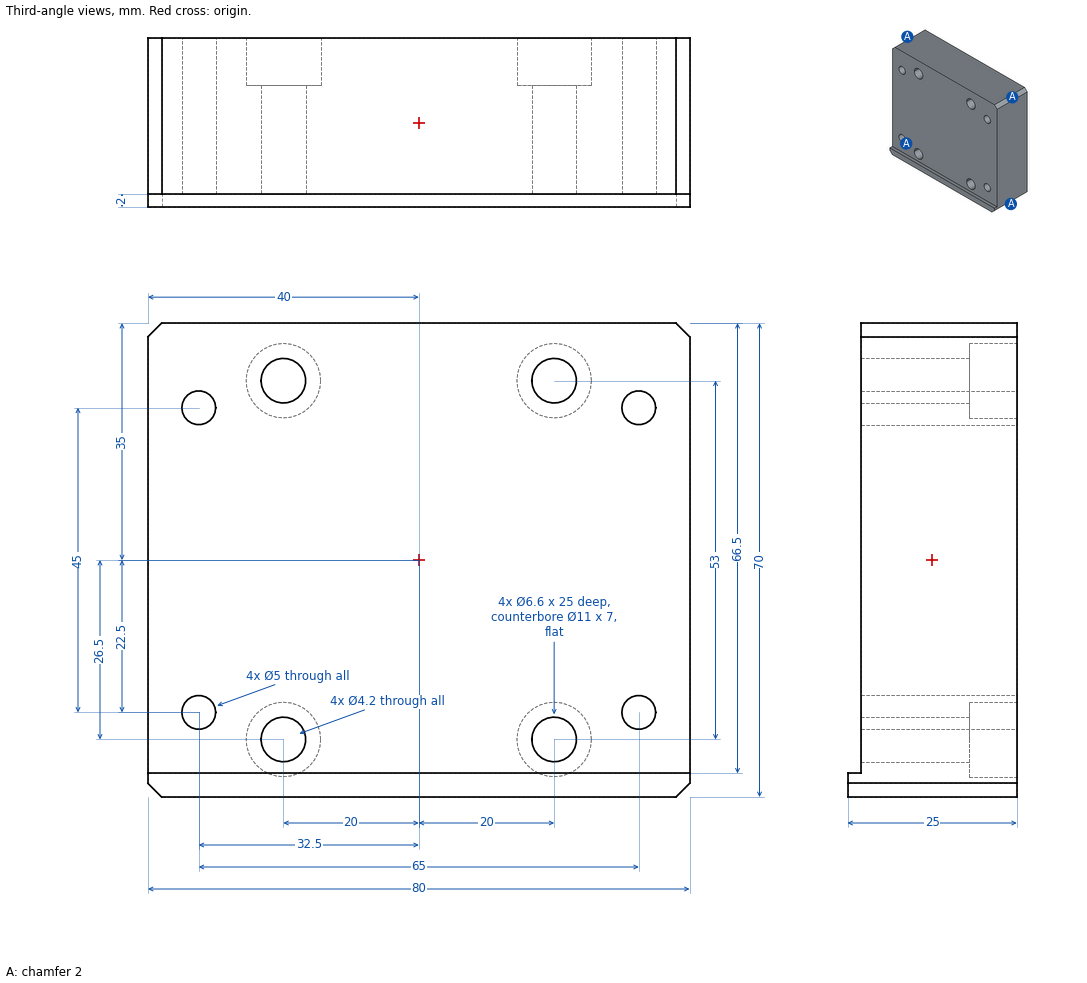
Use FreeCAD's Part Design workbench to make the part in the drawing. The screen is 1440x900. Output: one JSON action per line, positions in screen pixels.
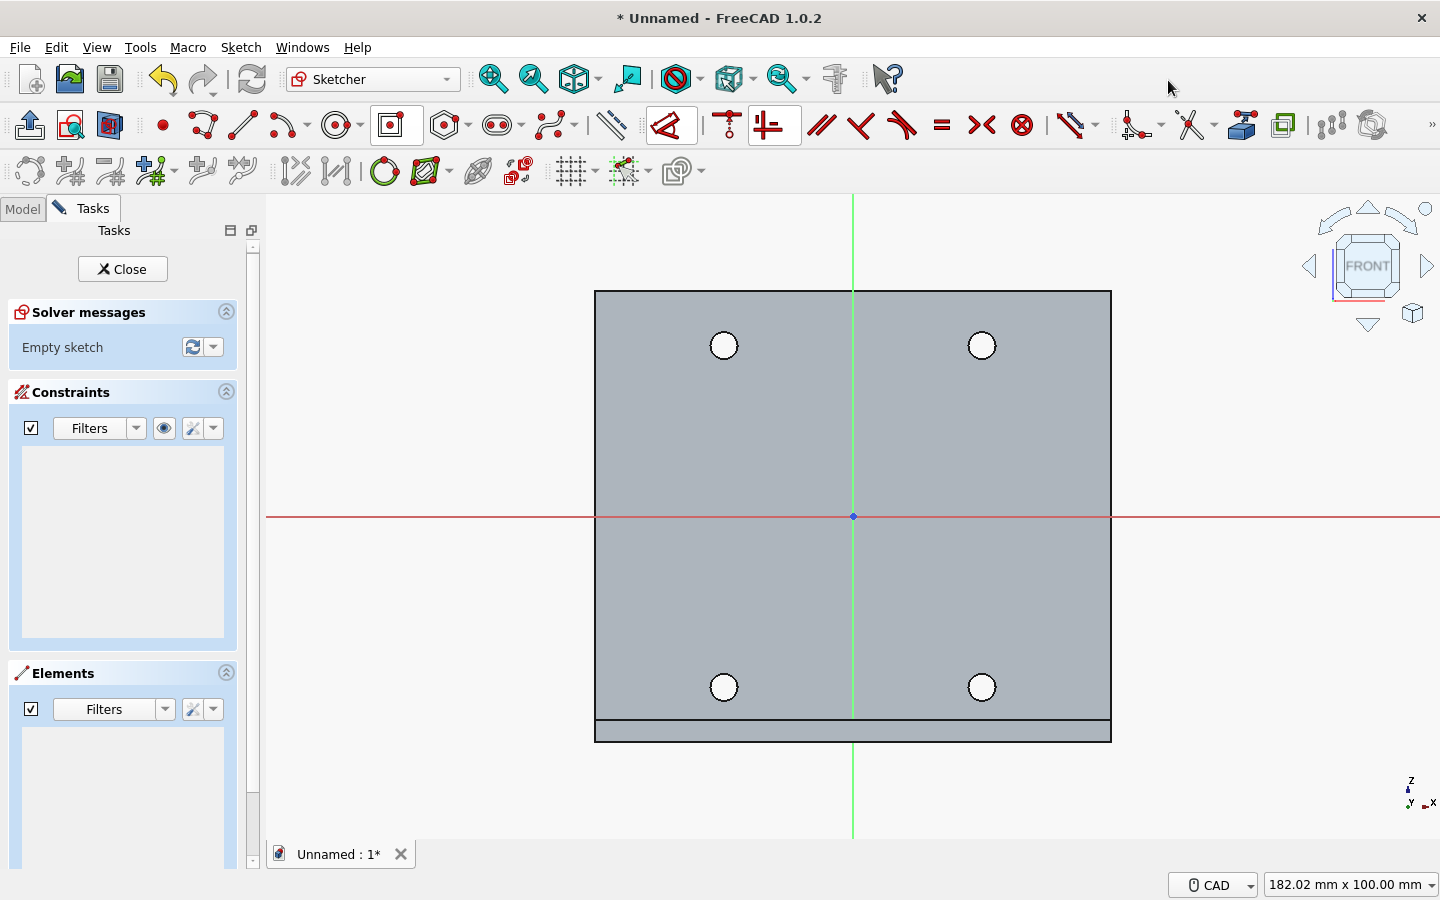
{"action": "left_click", "coordinate": [110, 126]}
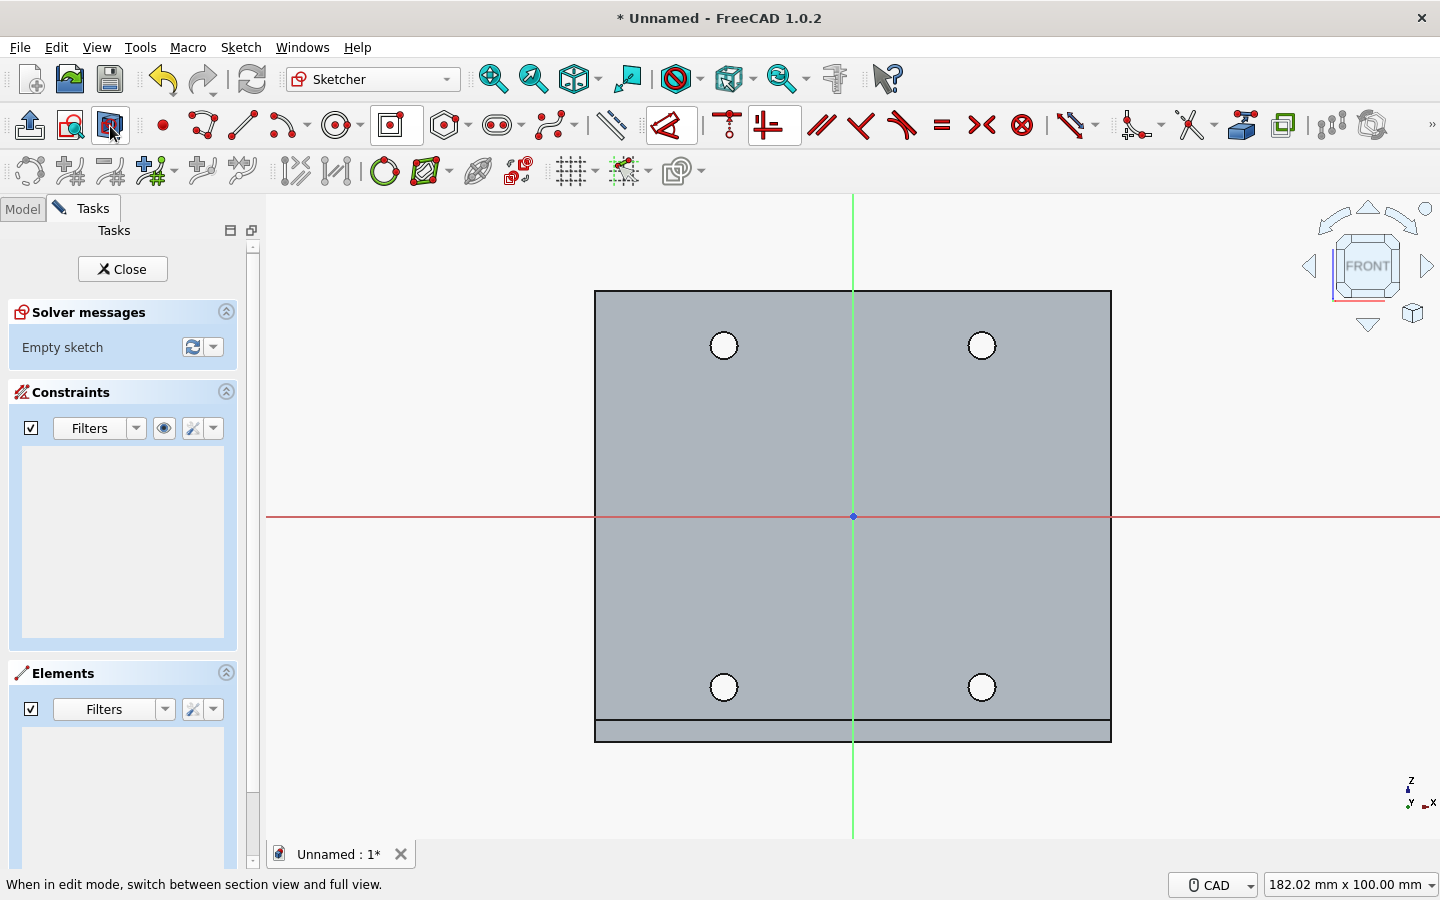
{"action": "left_click", "coordinate": [336, 126]}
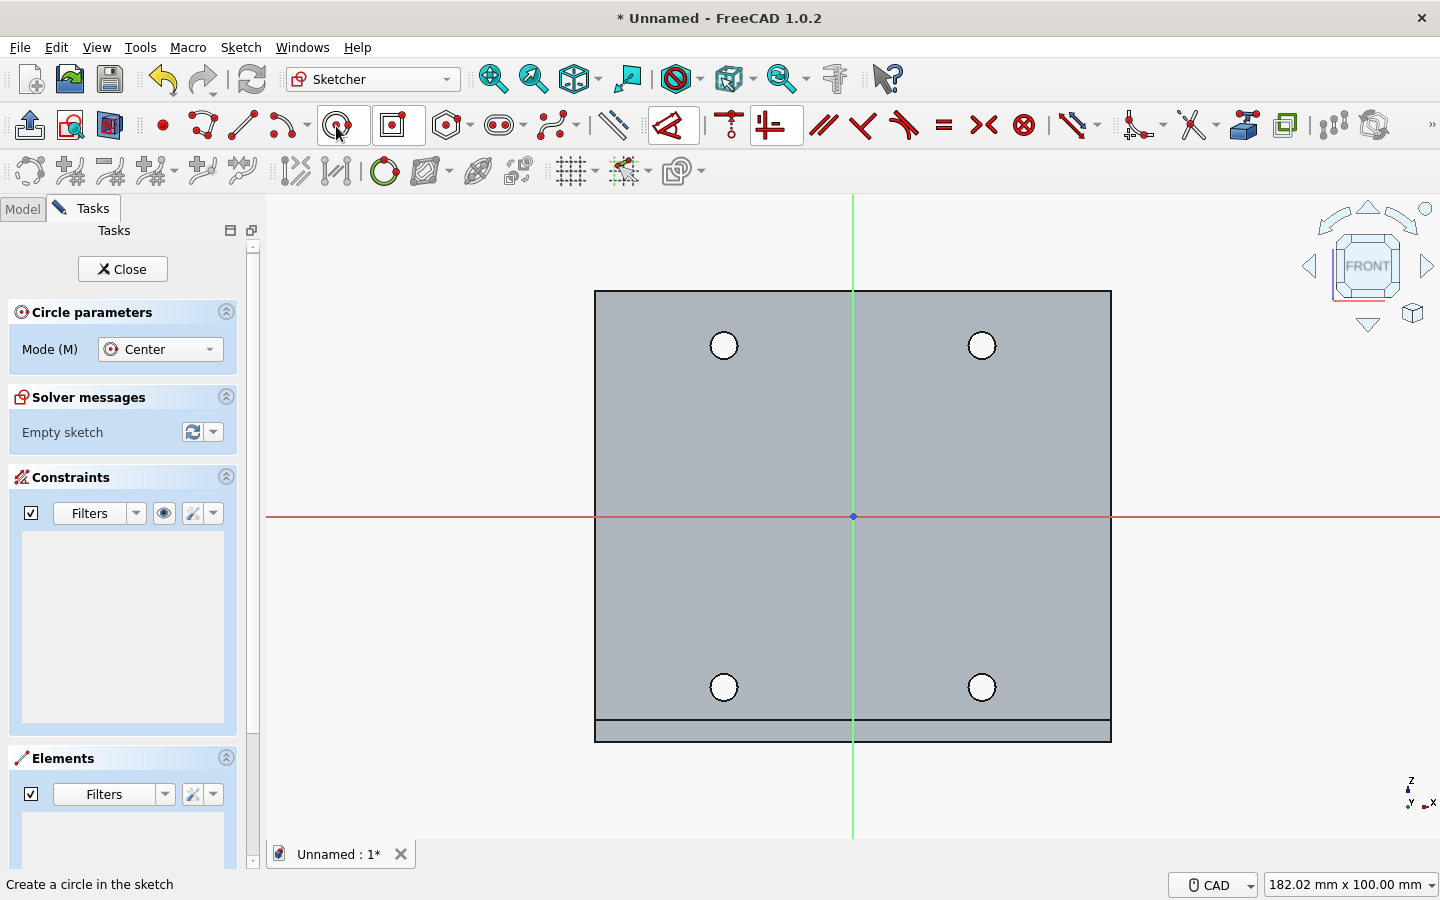
{"action": "scroll", "coordinate": [643, 662], "scroll_direction": "up", "scroll_amount": 2}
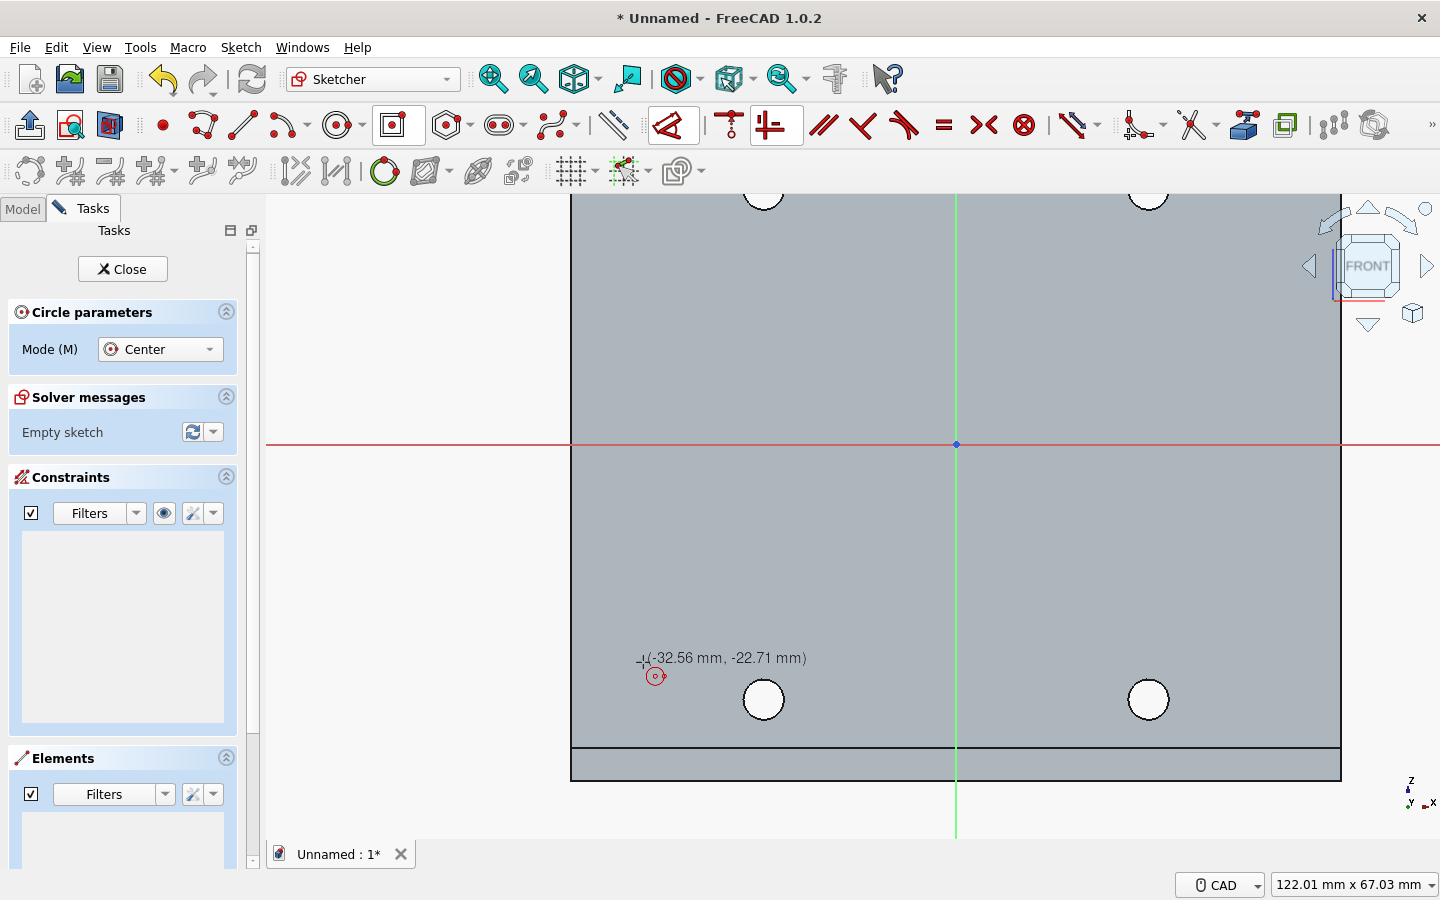
{"action": "left_click", "coordinate": [643, 661]}
{"action": "mouse_move", "coordinate": [660, 644]}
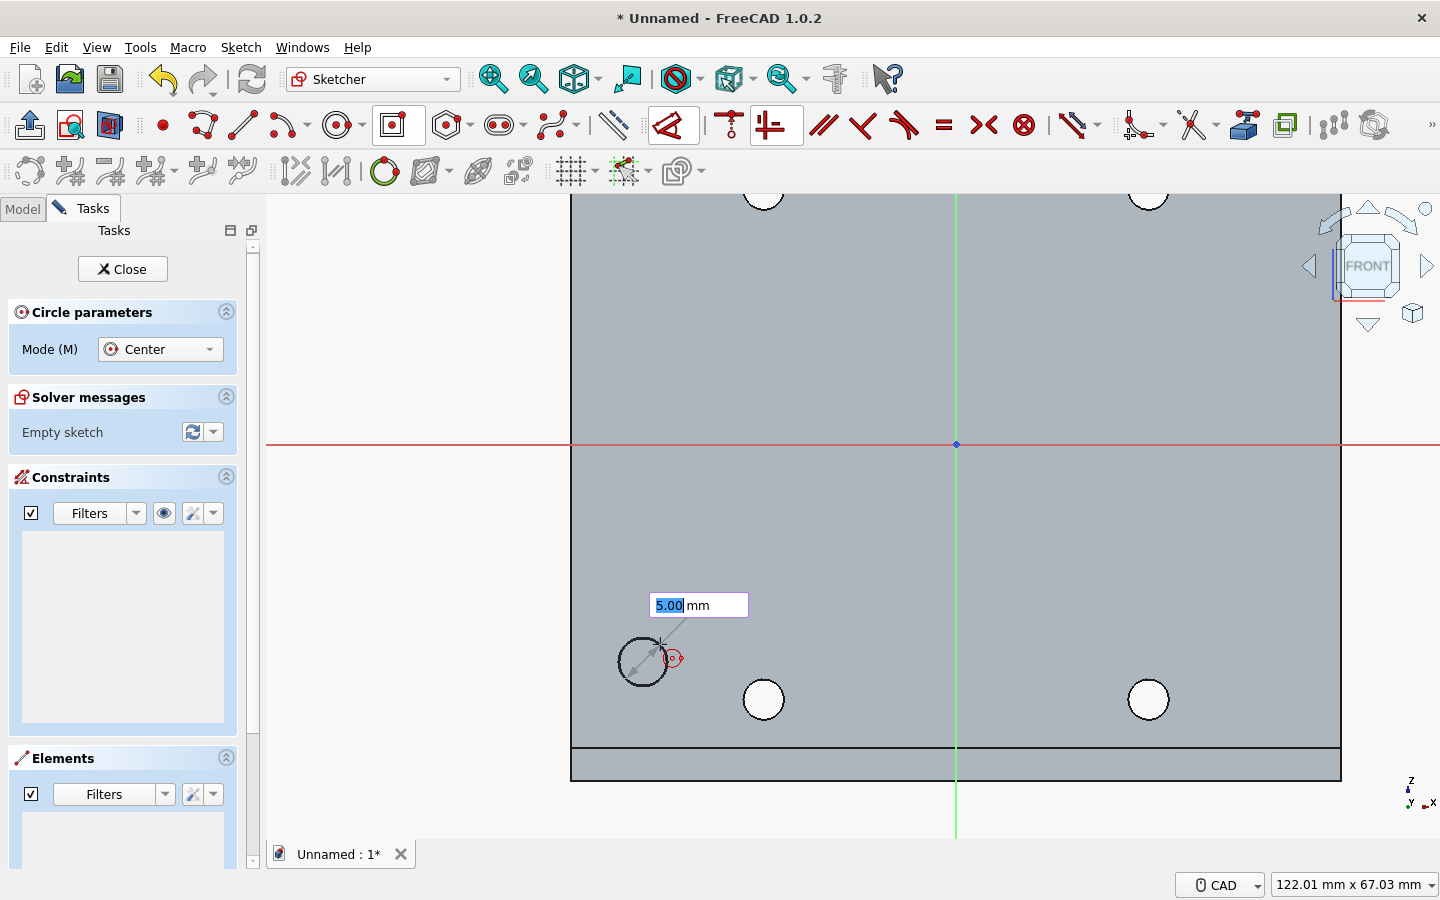
{"action": "type", "text": "5"}
{"action": "key", "text": "Return"}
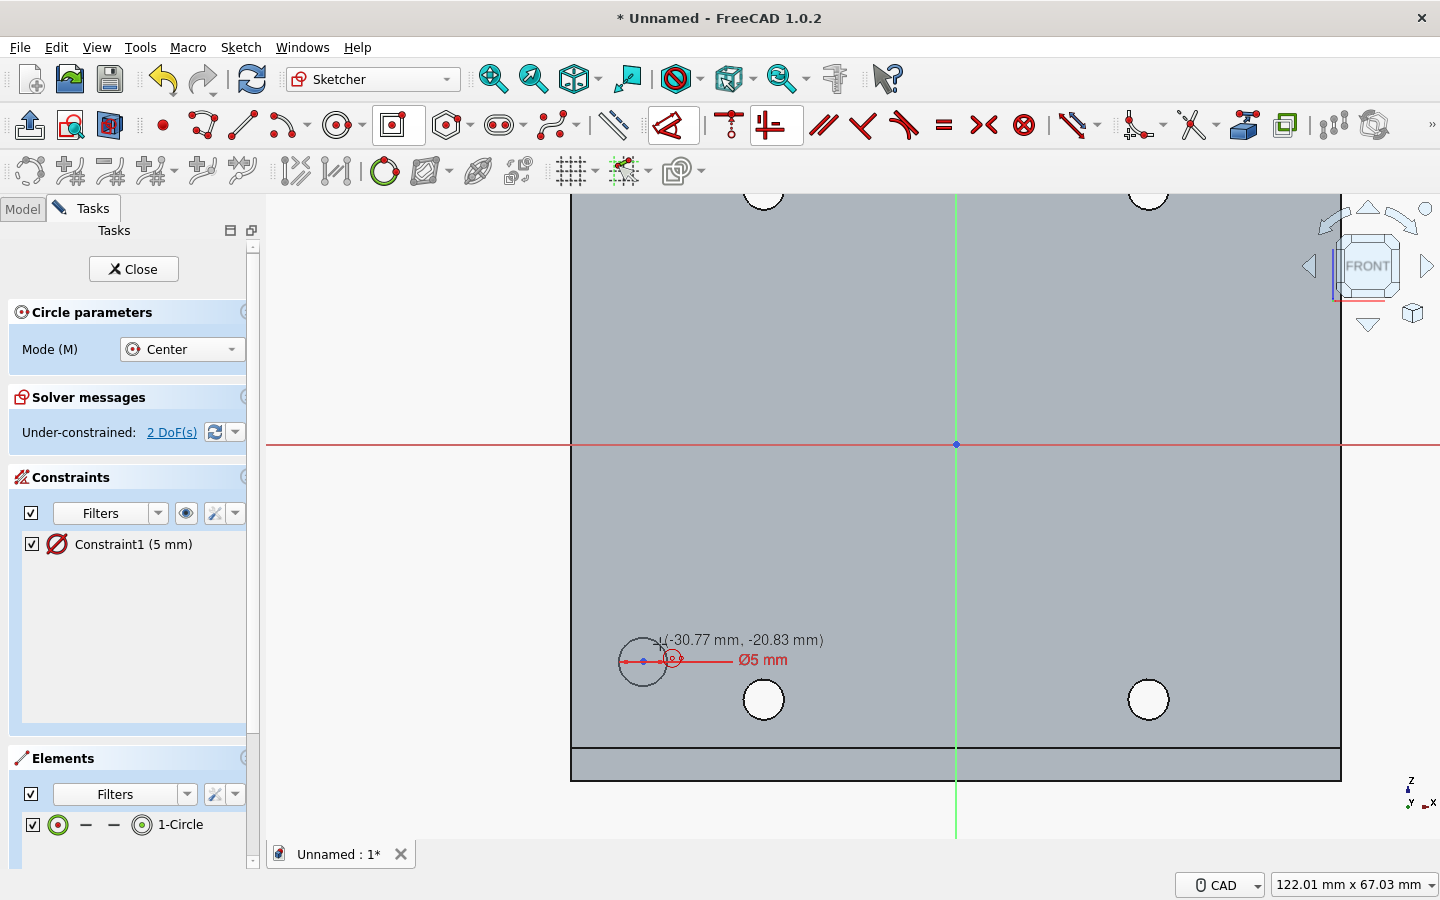
{"action": "left_click", "coordinate": [643, 228]}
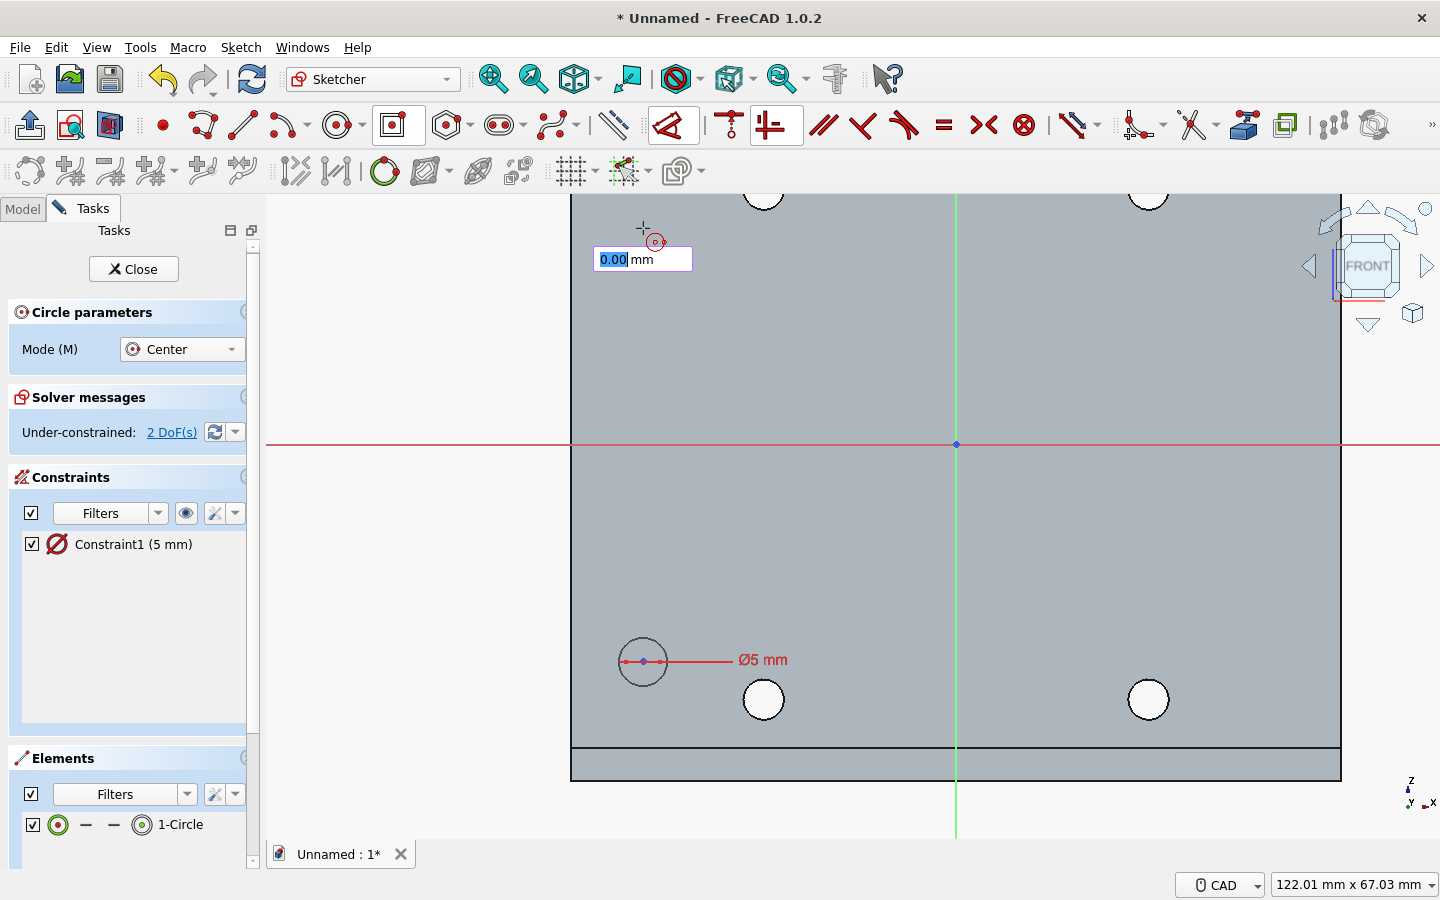
{"action": "scroll", "coordinate": [294, 811], "scroll_direction": "down", "scroll_amount": 1}
{"action": "mouse_move", "coordinate": [594, 320]}